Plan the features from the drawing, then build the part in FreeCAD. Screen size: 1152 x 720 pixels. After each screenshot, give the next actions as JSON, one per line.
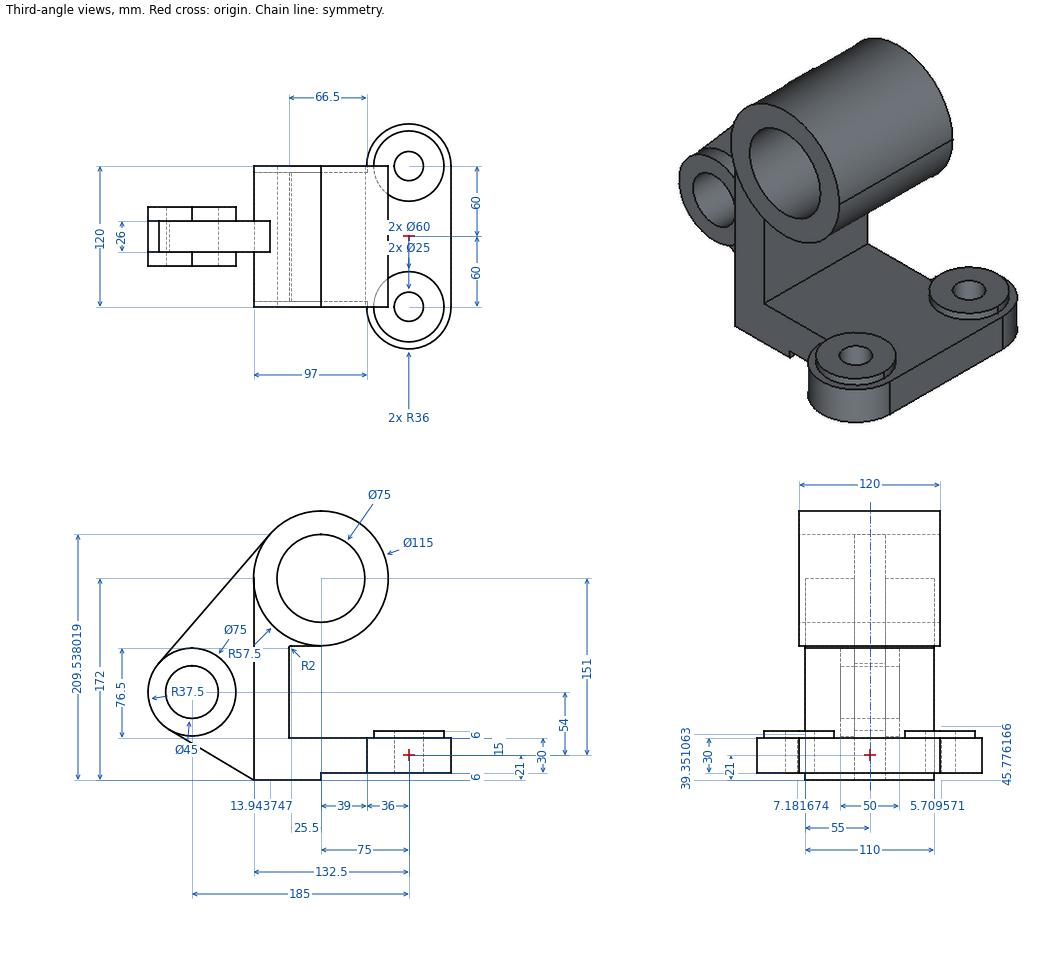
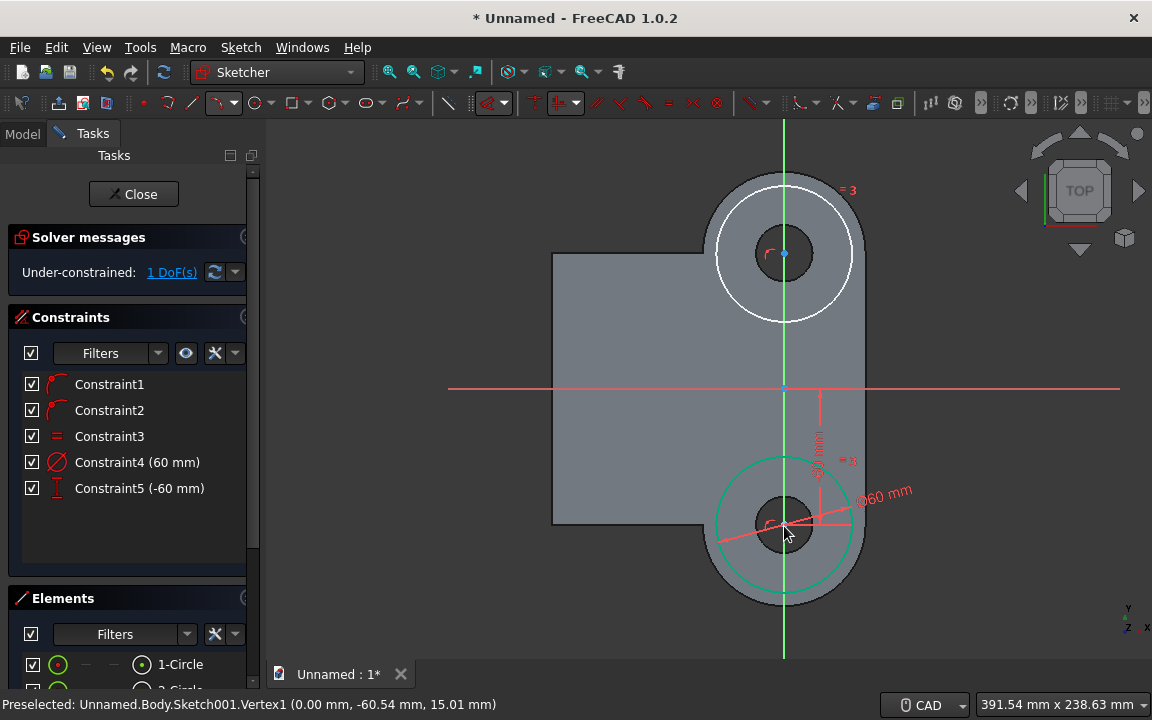
{"action": "left_click", "coordinate": [784, 254]}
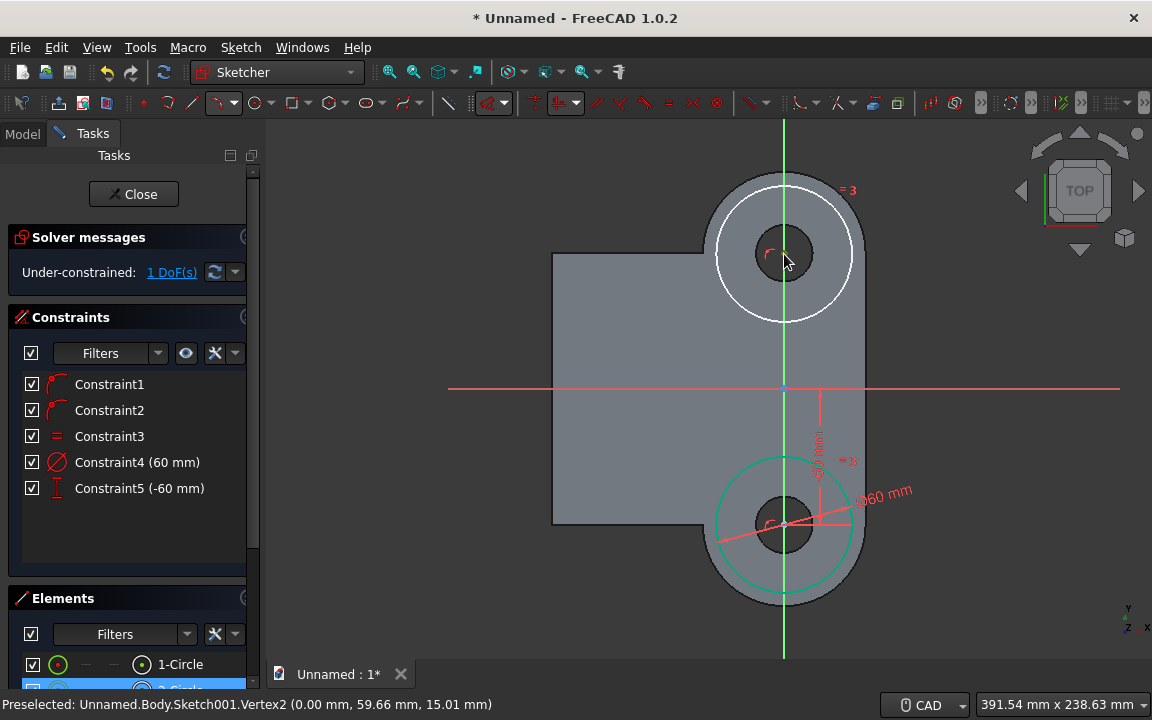
{"action": "key", "text": "i"}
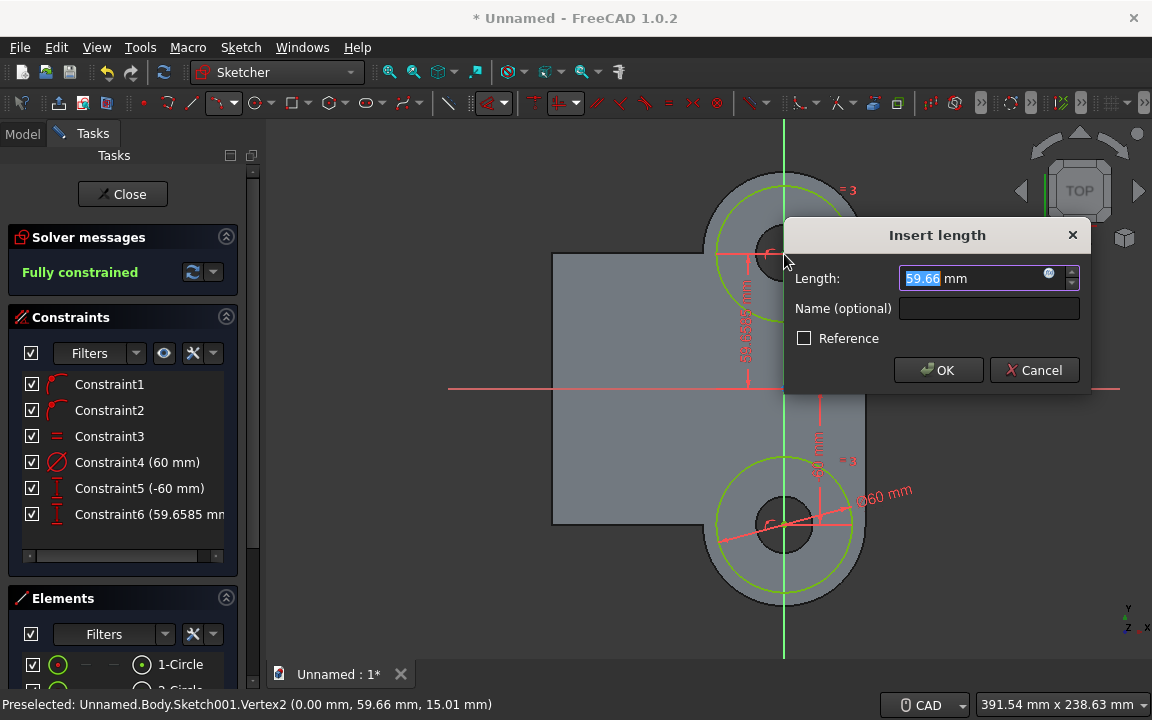
{"action": "type", "text": "60"}
{"action": "key", "text": "Return"}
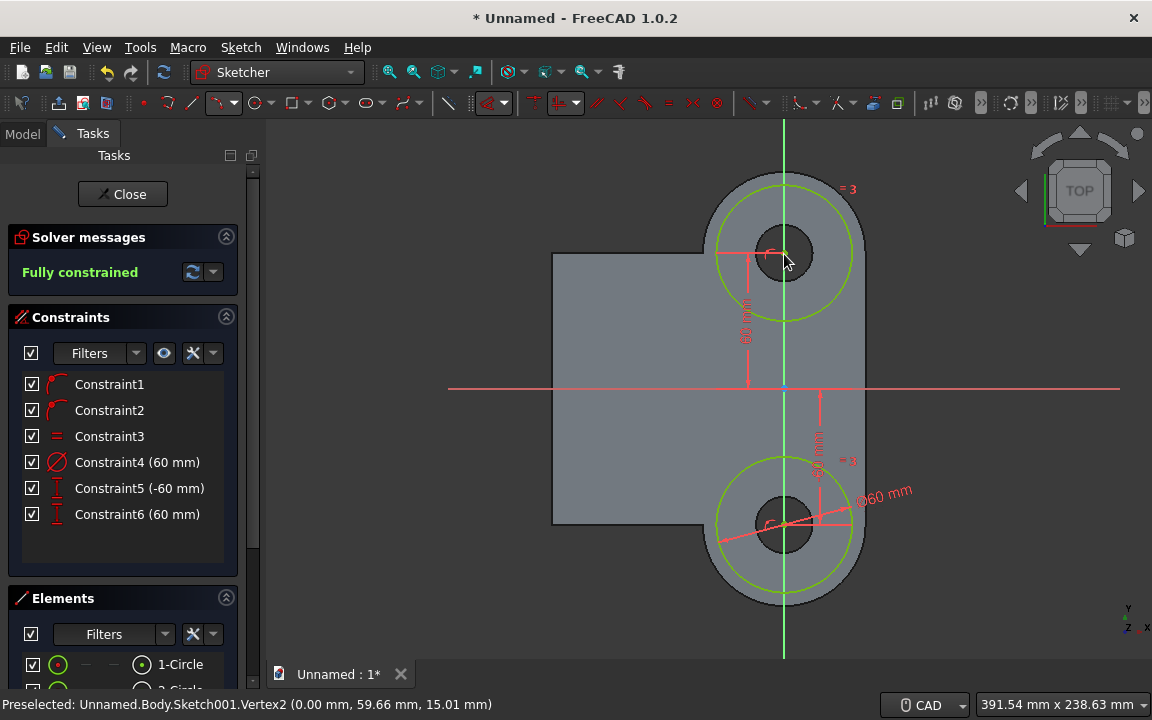
{"action": "left_click", "coordinate": [123, 194]}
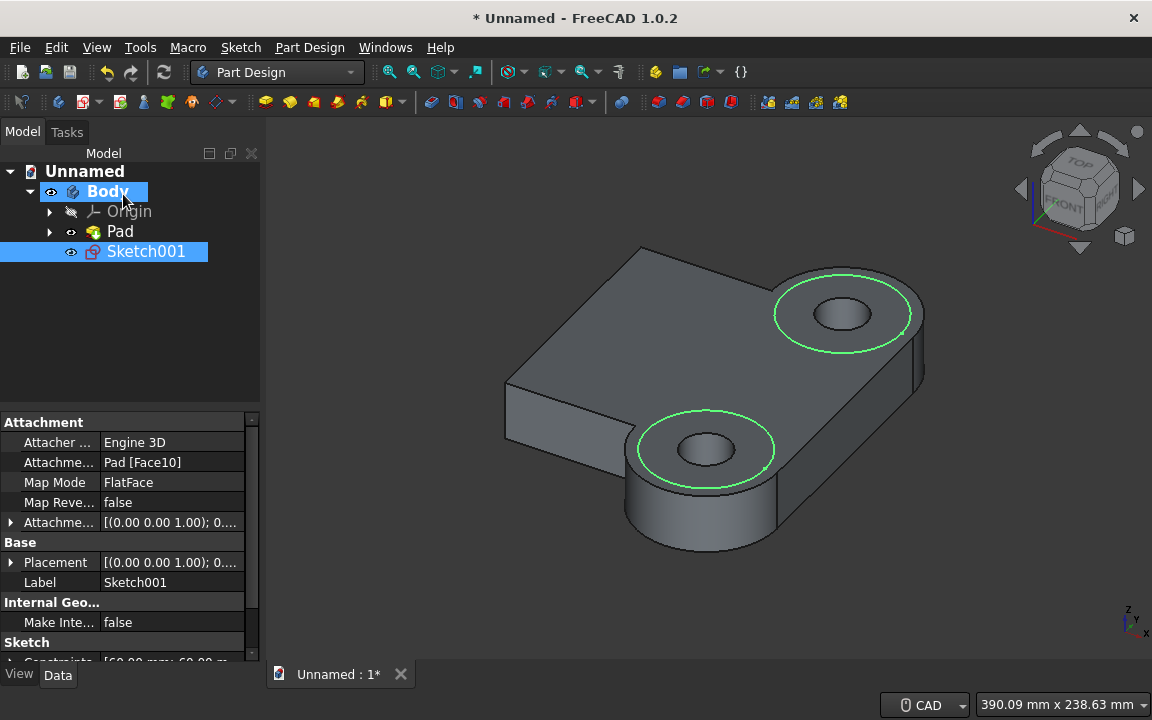
{"action": "left_click", "coordinate": [266, 102]}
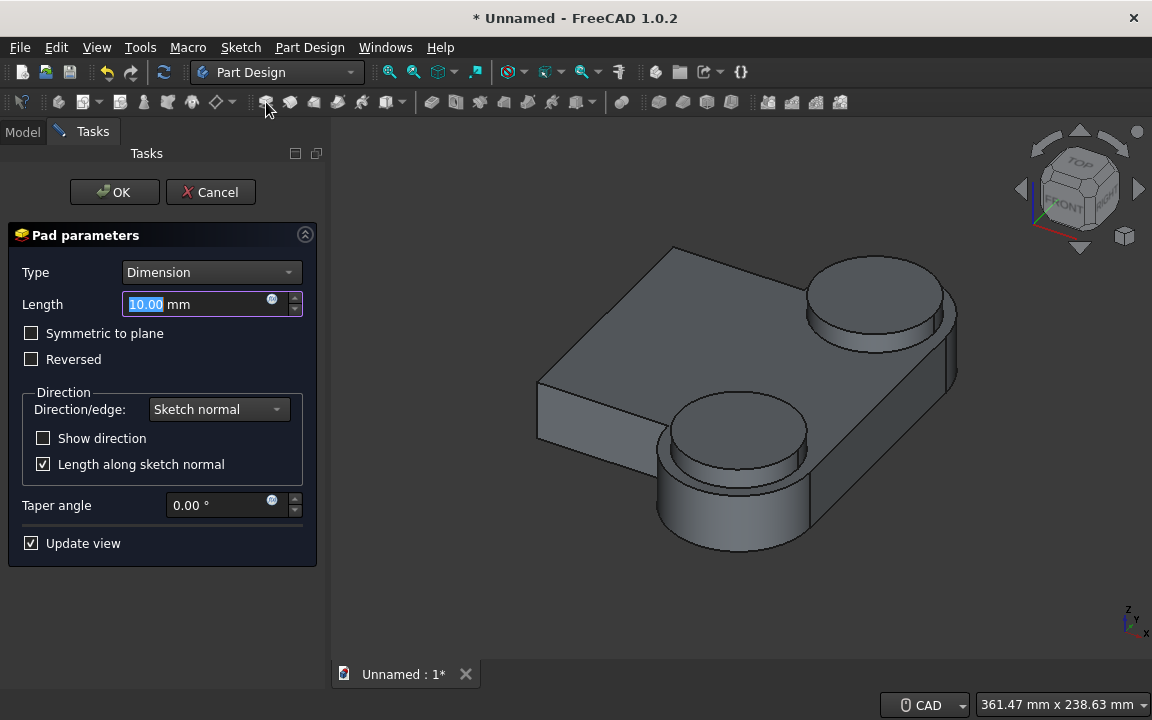
{"action": "type", "text": "6"}
{"action": "key", "text": "Tab"}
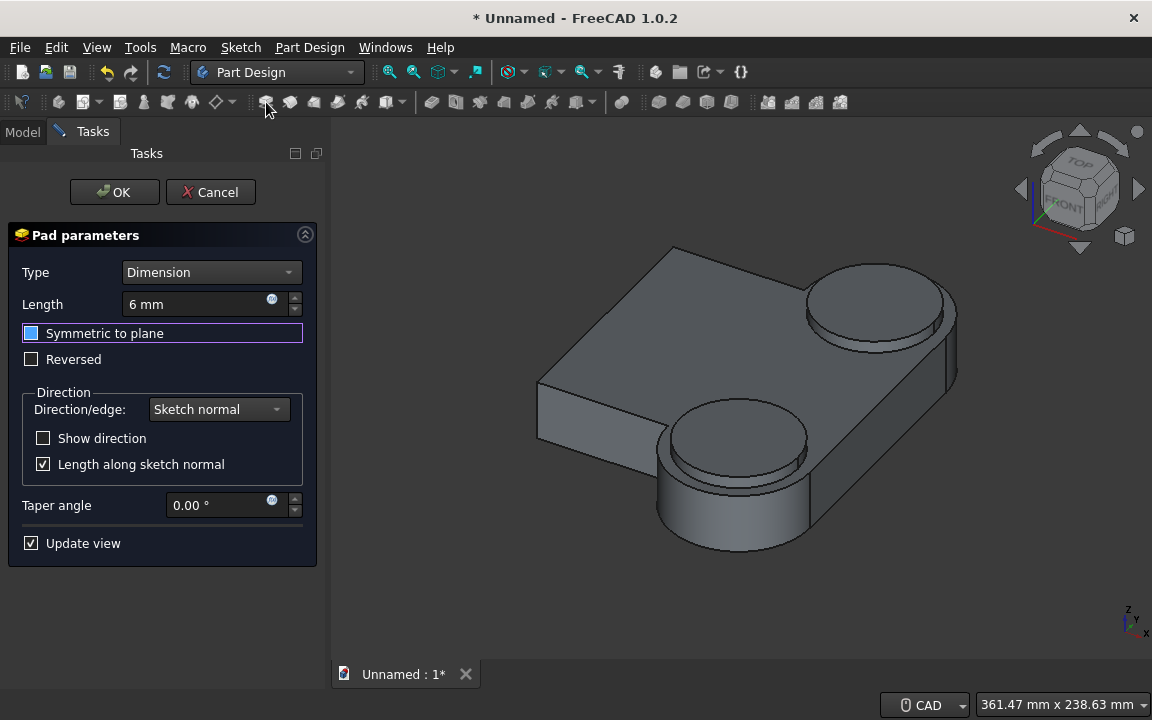
{"action": "left_click", "coordinate": [115, 192]}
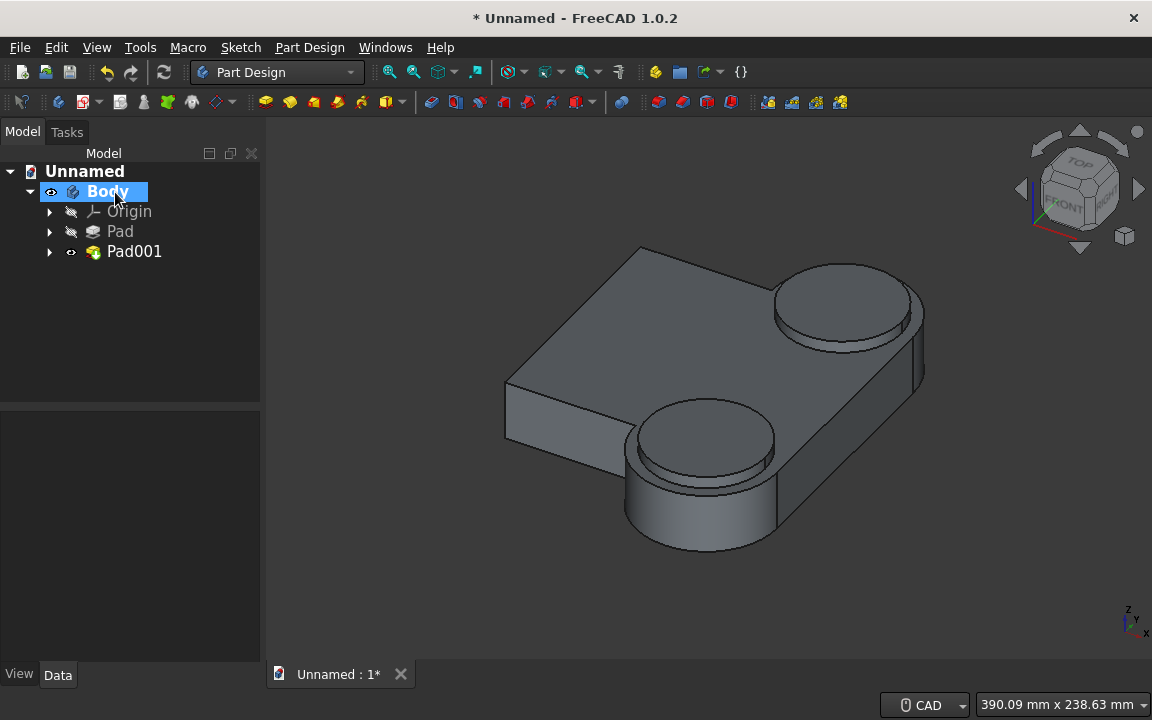
{"action": "key", "text": "5"}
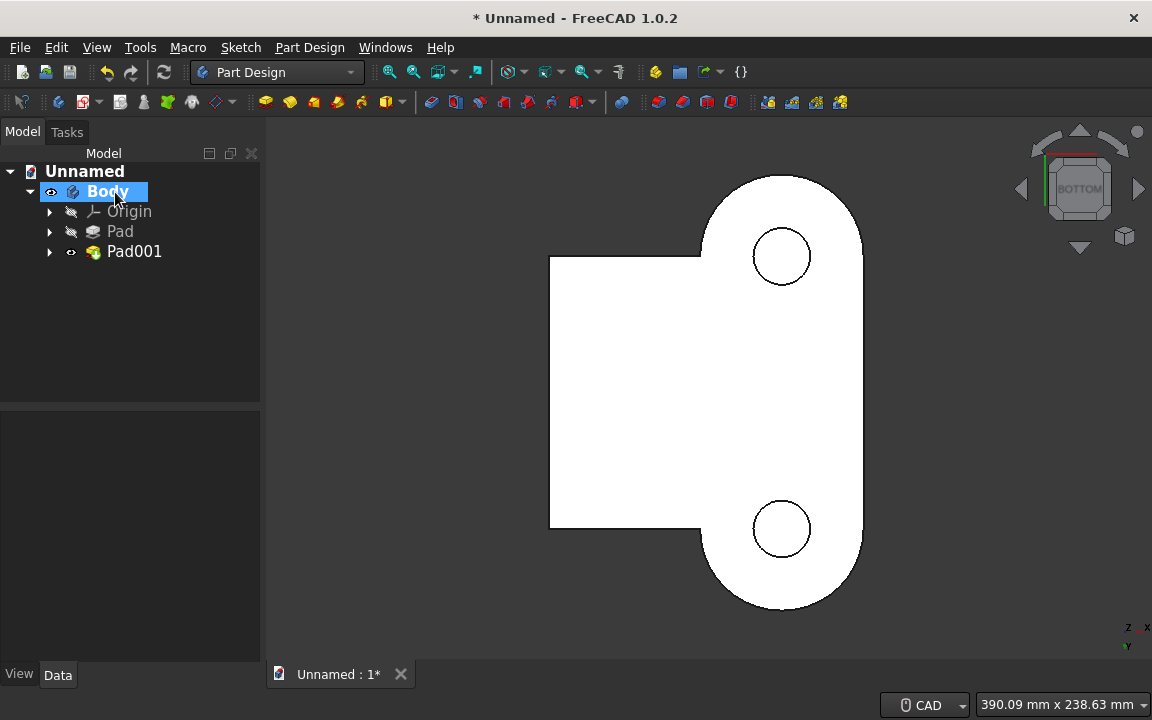
{"action": "left_click", "coordinate": [706, 392]}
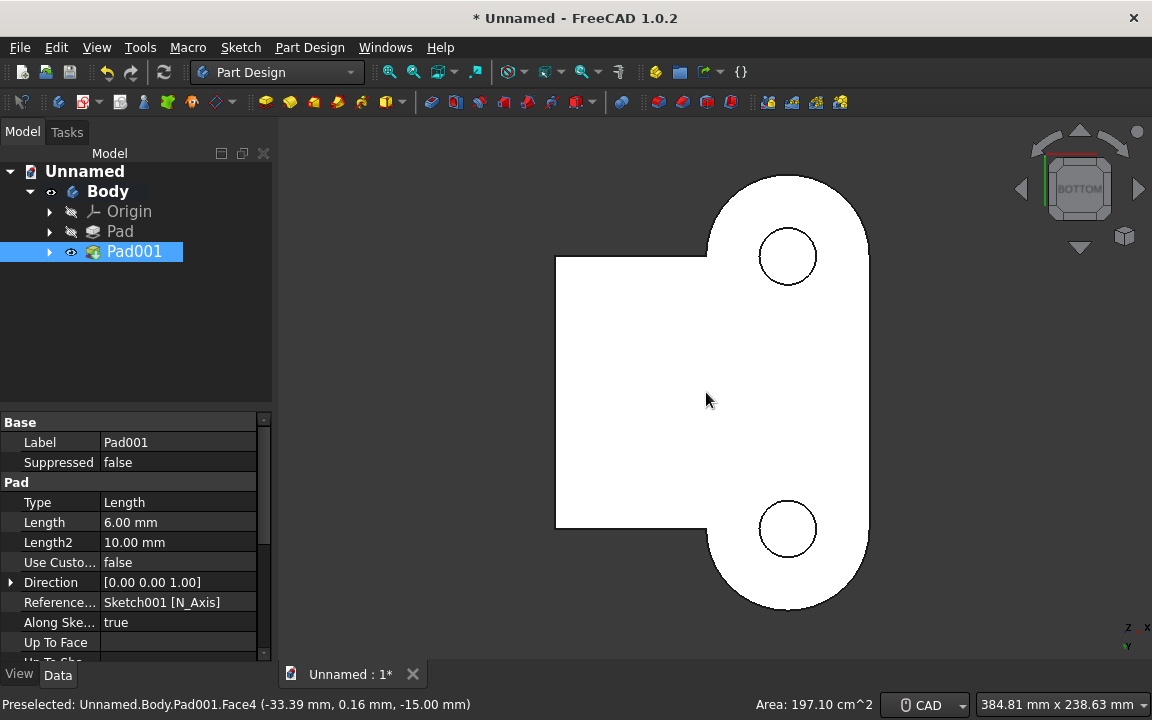
{"action": "left_click", "coordinate": [84, 102]}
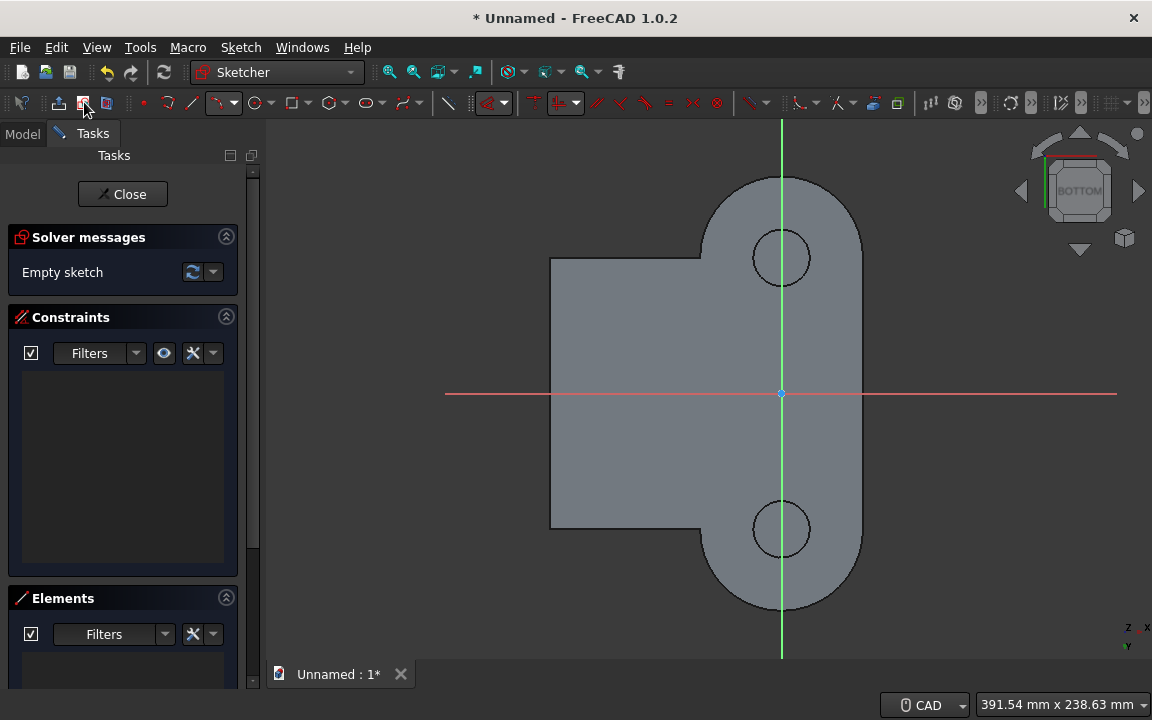
{"action": "key", "text": "g c"}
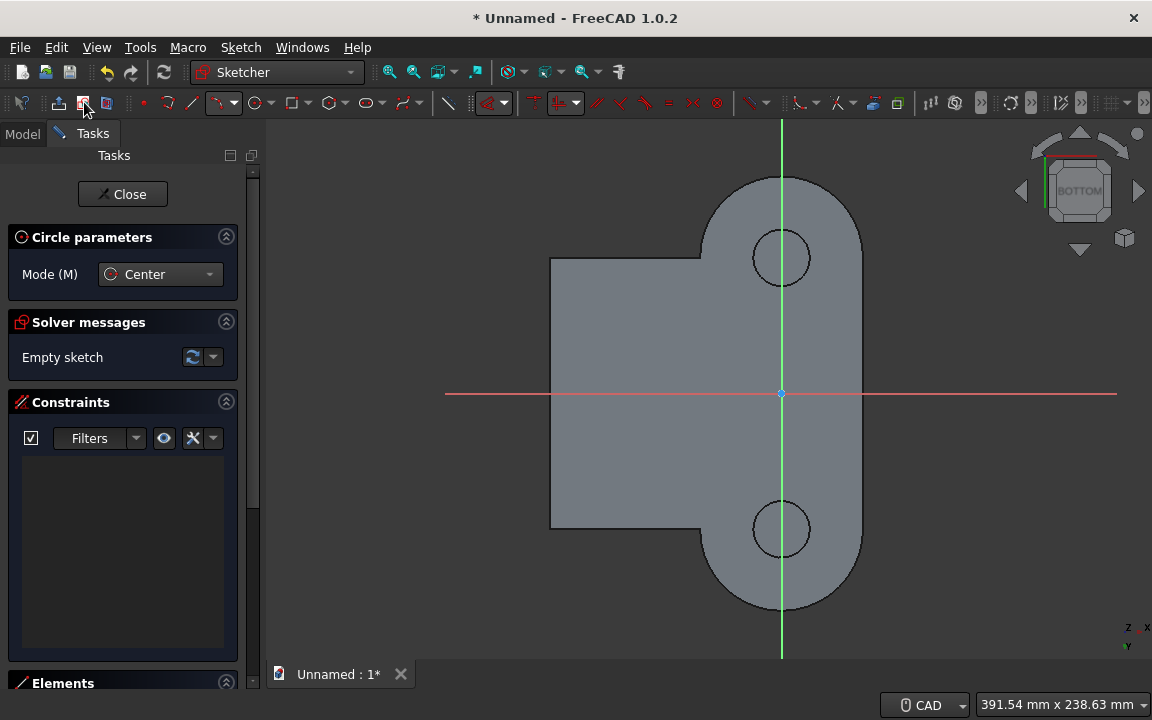
{"action": "left_click", "coordinate": [782, 258]}
{"action": "left_click", "coordinate": [802, 238]}